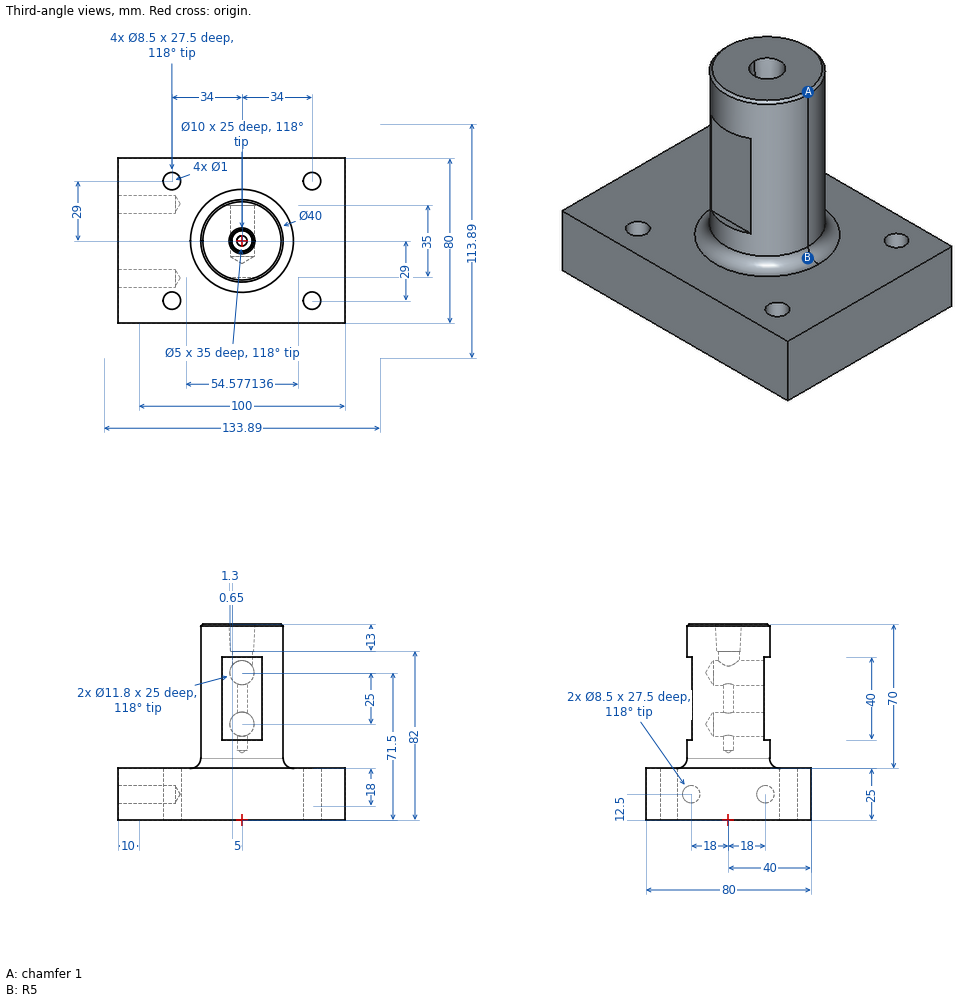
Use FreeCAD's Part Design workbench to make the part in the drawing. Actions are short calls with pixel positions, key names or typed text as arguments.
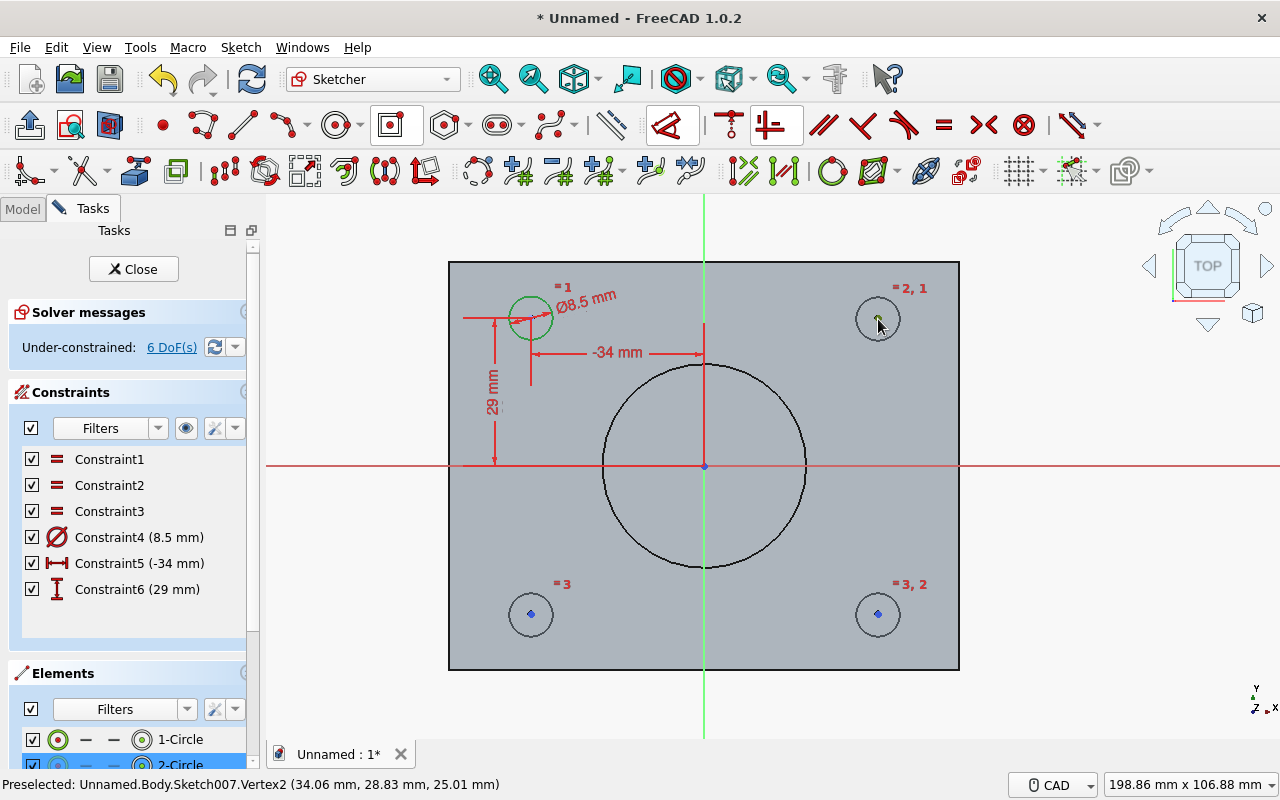
key(l)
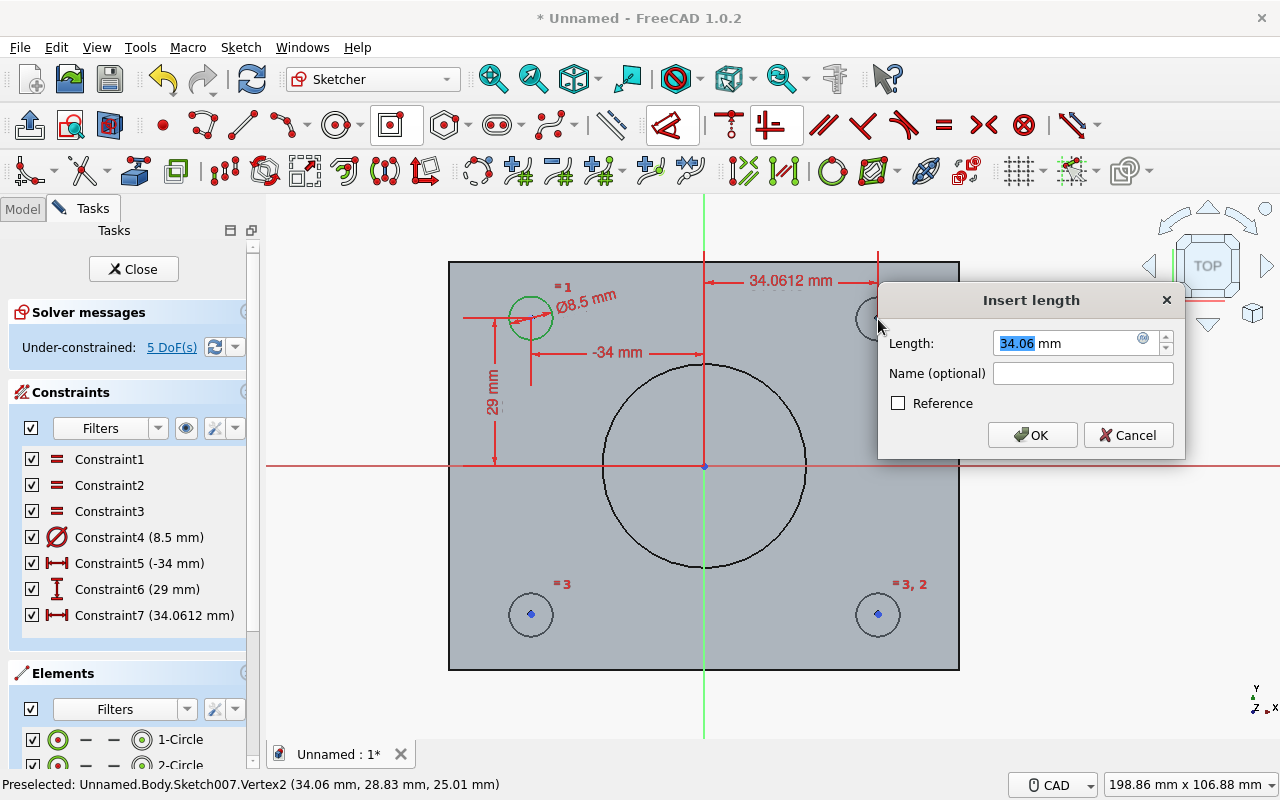
text(34)
key(Return)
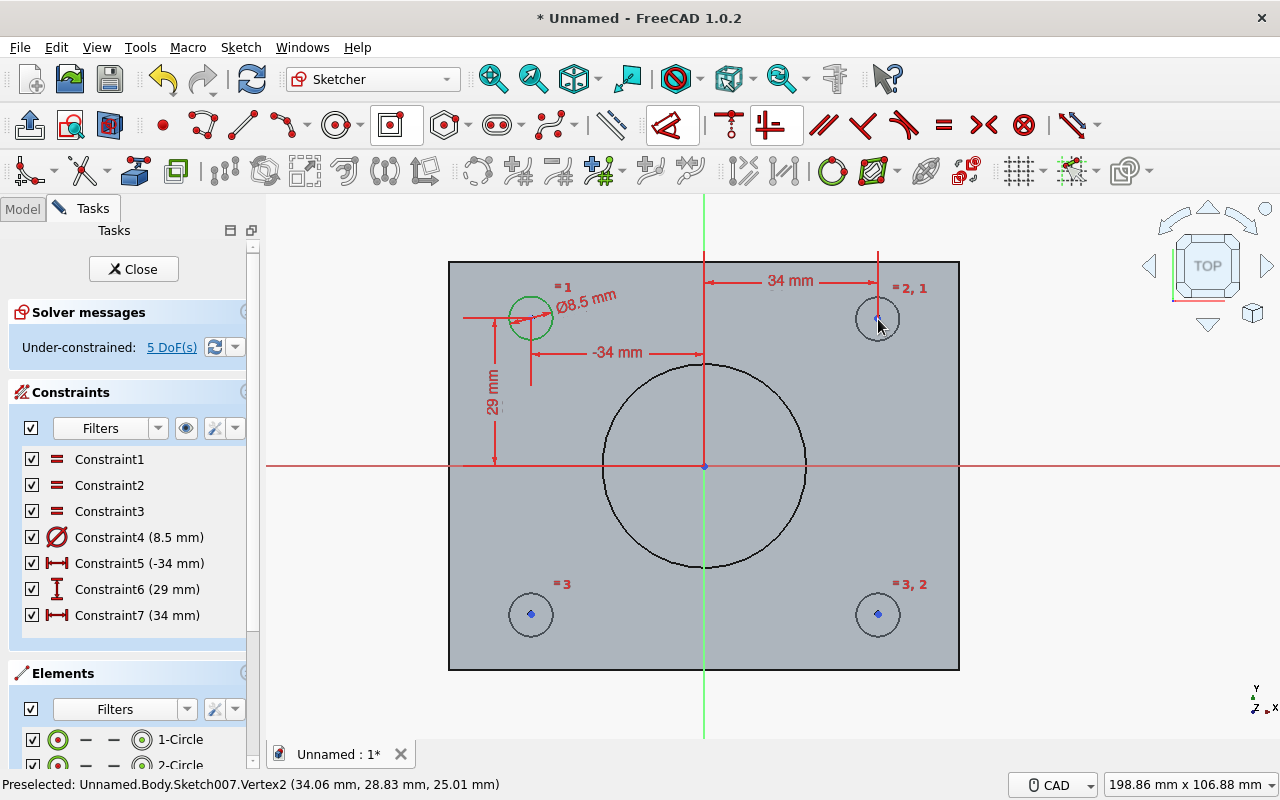
click(878, 319)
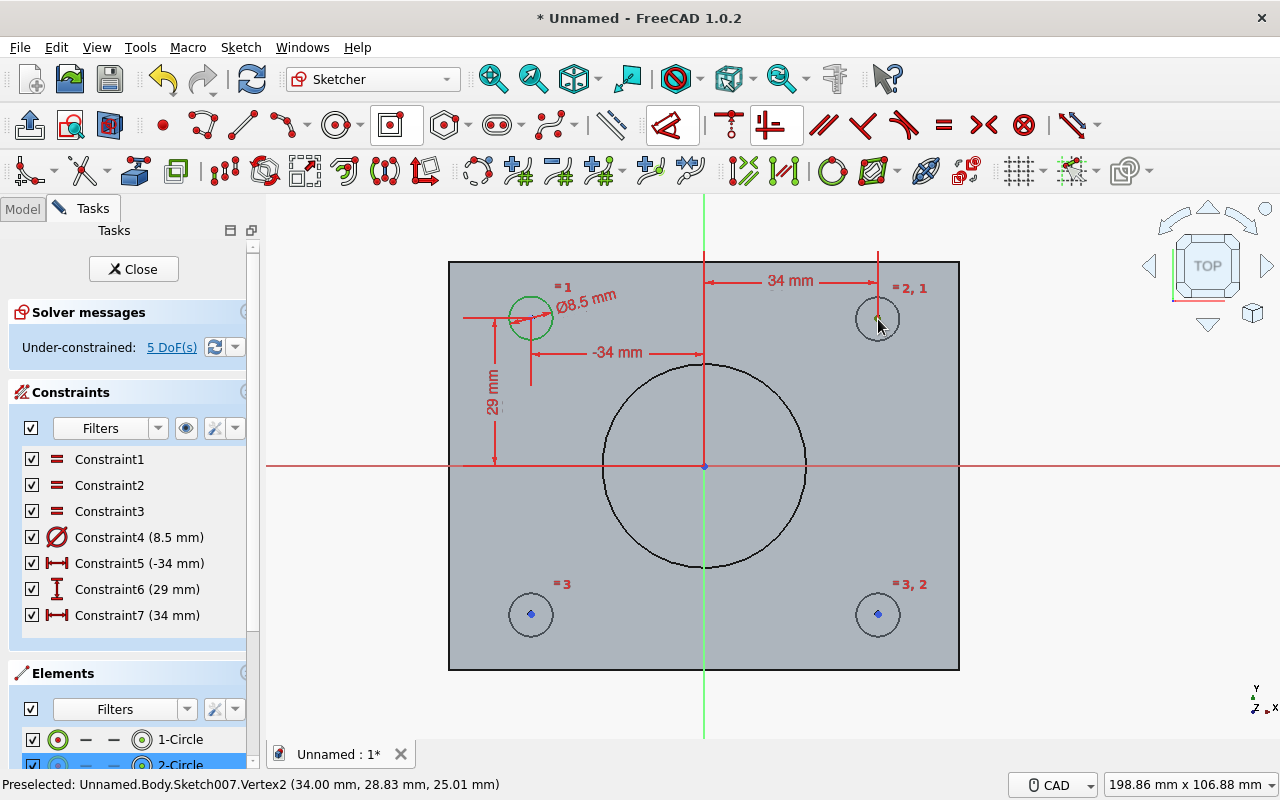
click(694, 126)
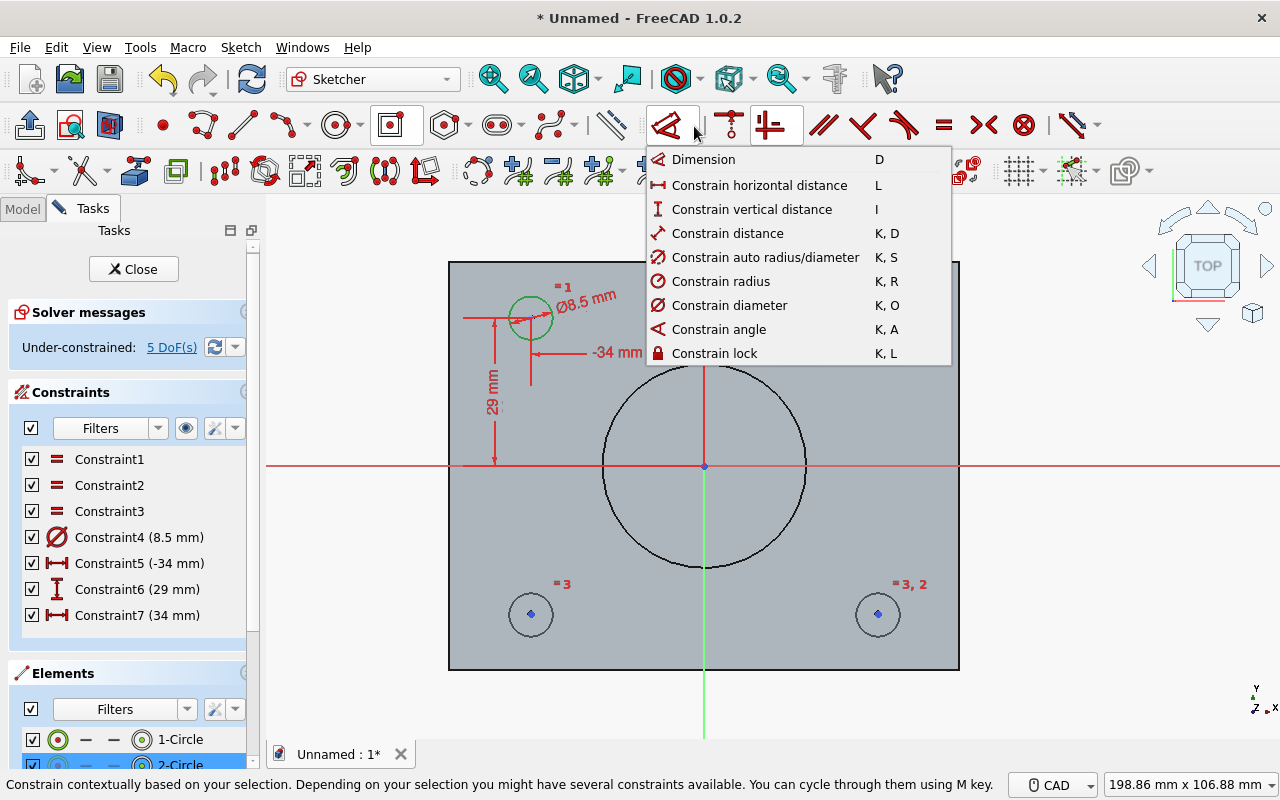
click(799, 209)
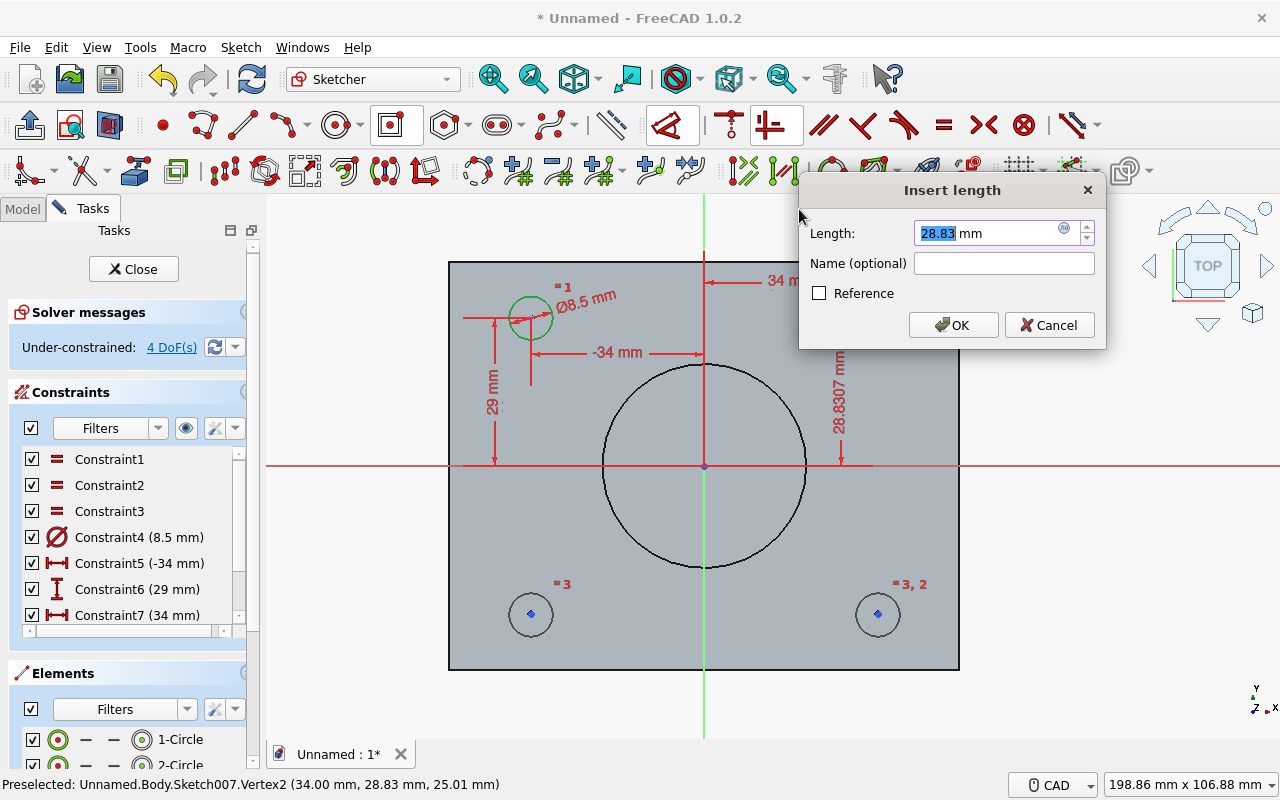
text(29)
key(Return)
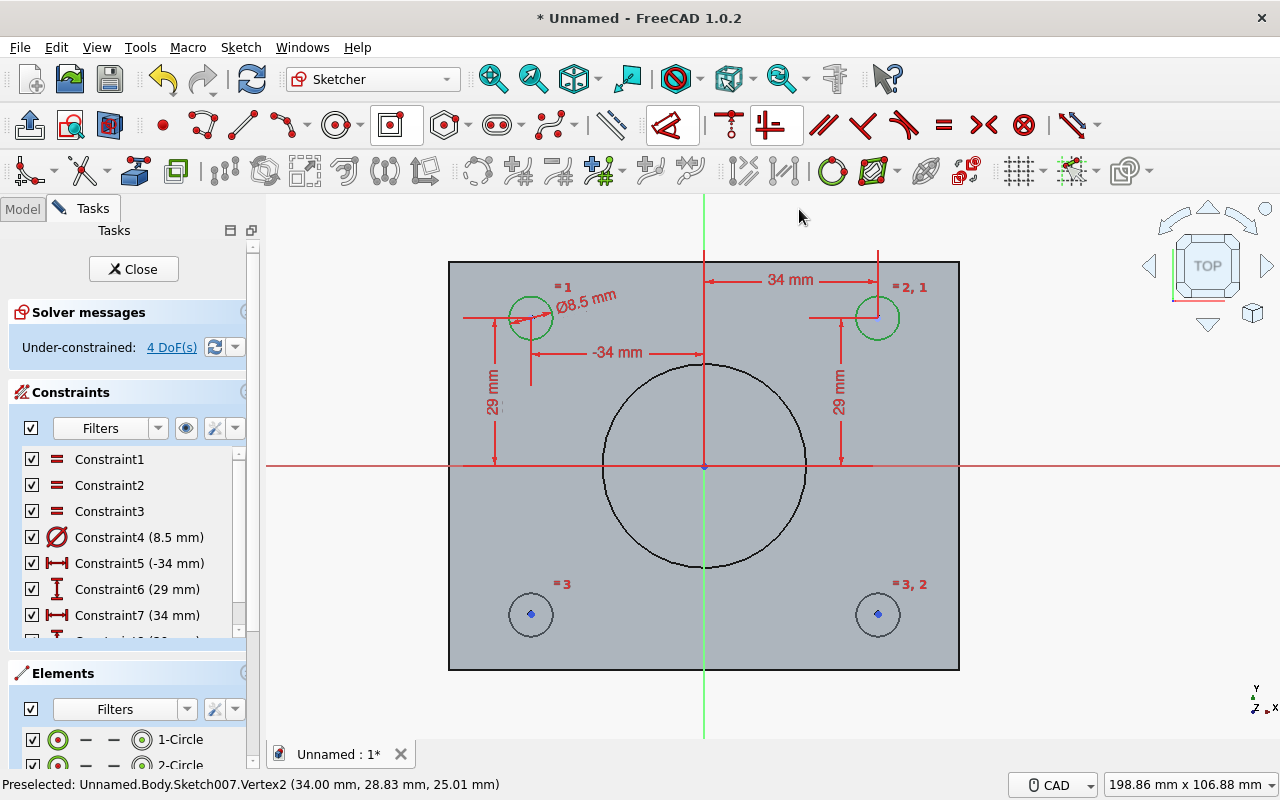
click(878, 615)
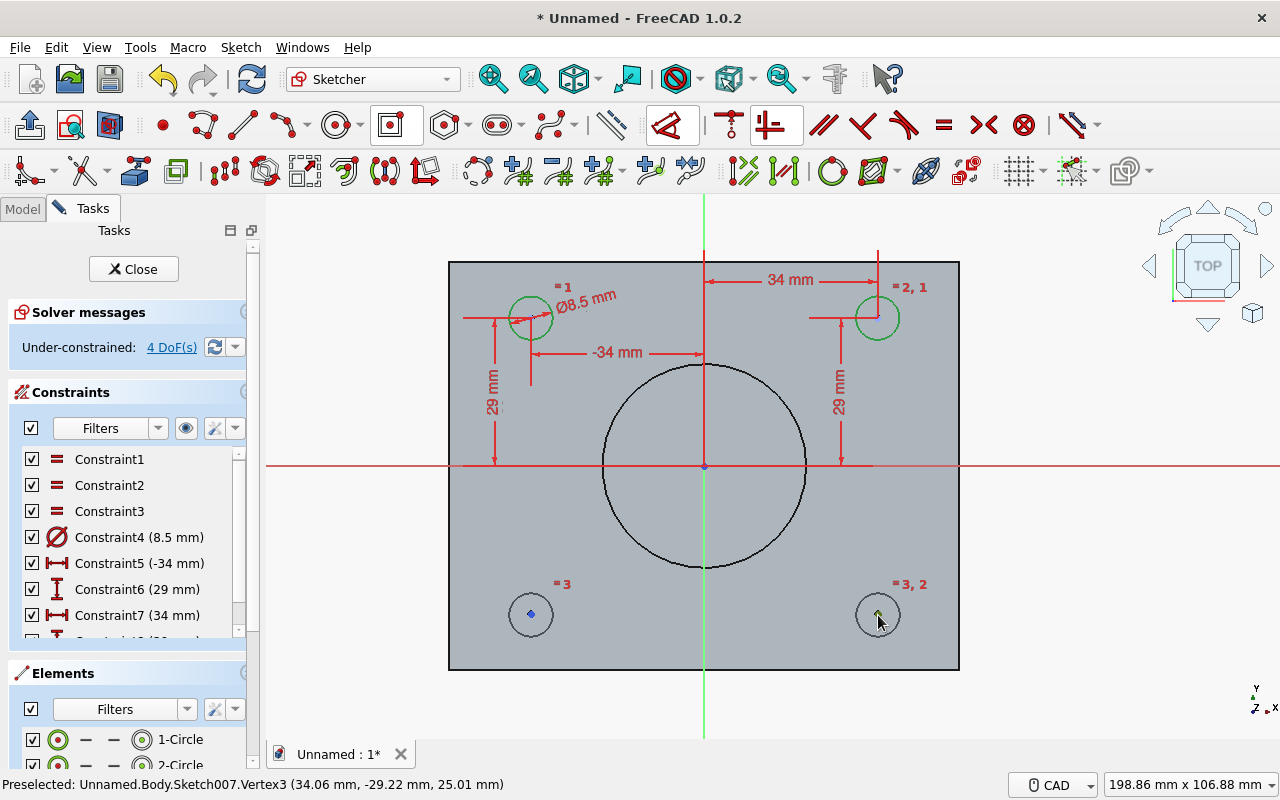
click(694, 126)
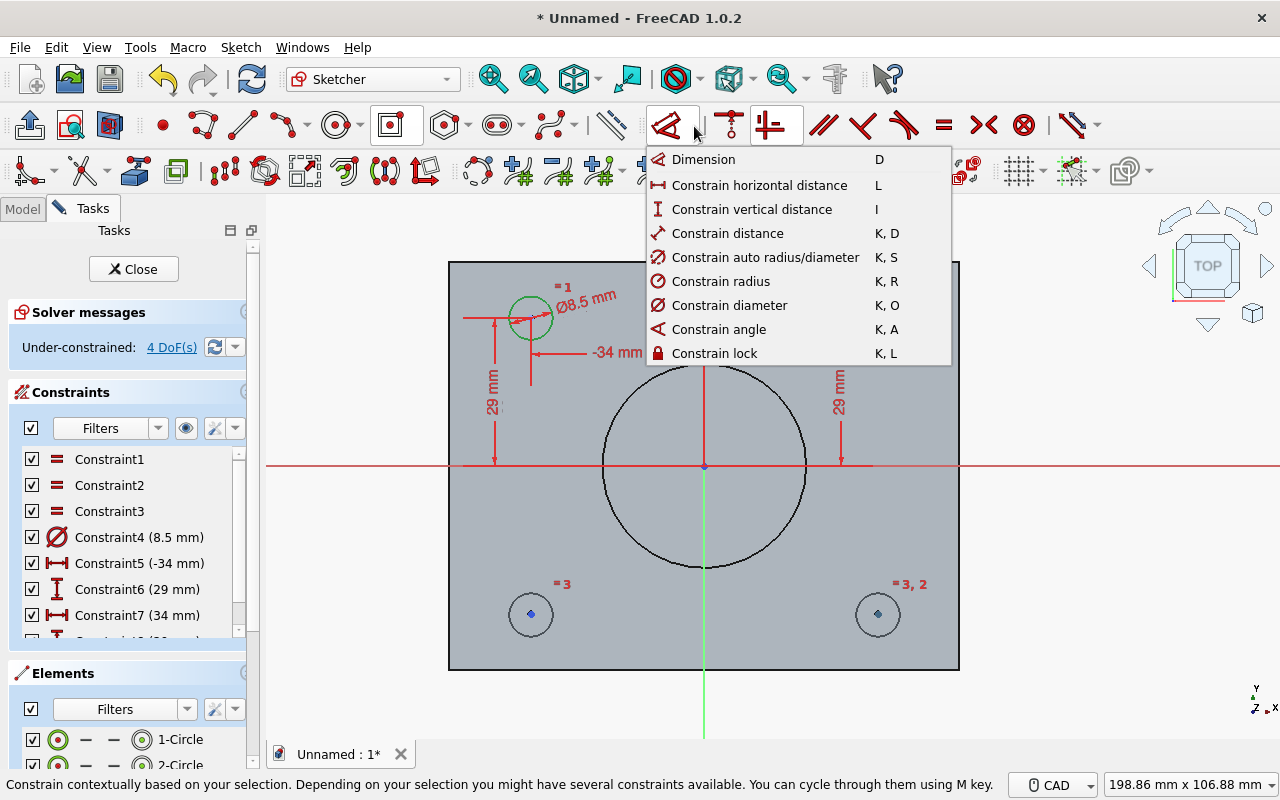
click(799, 185)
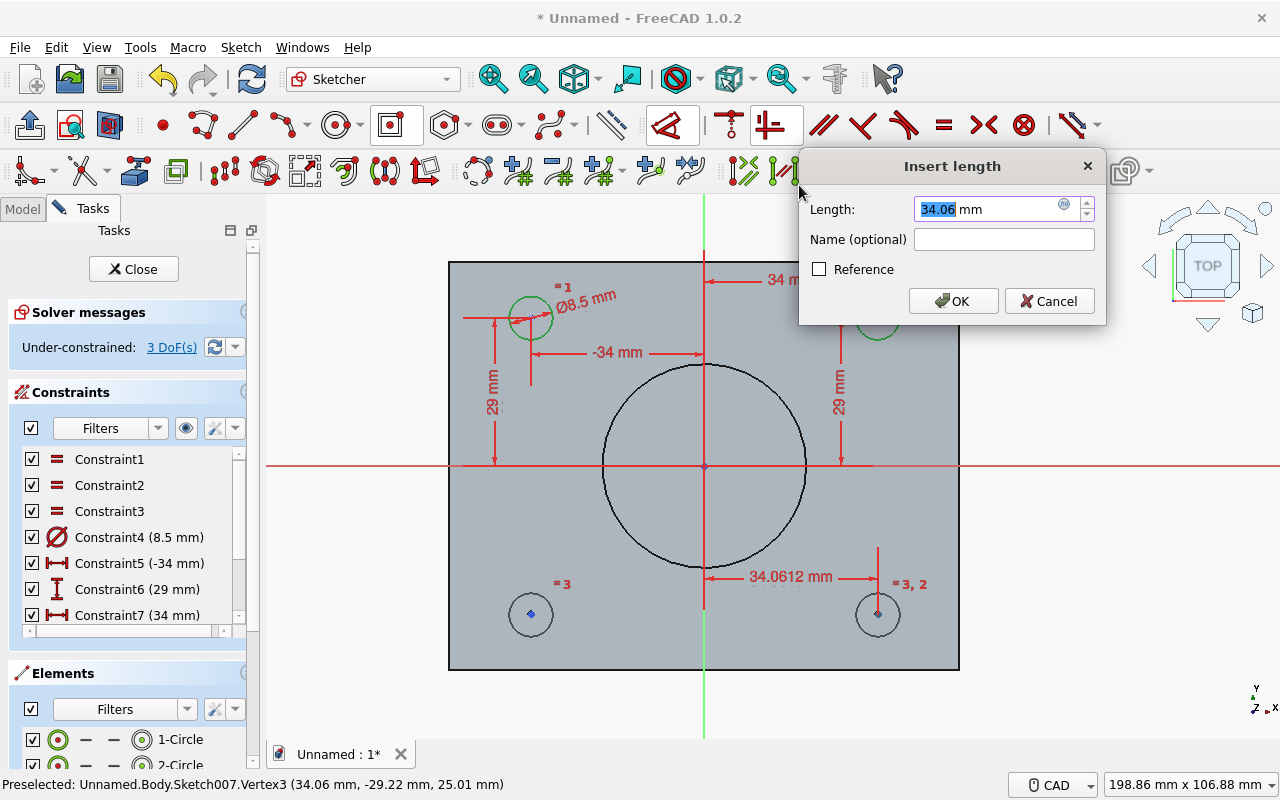
text(34)
key(Return)